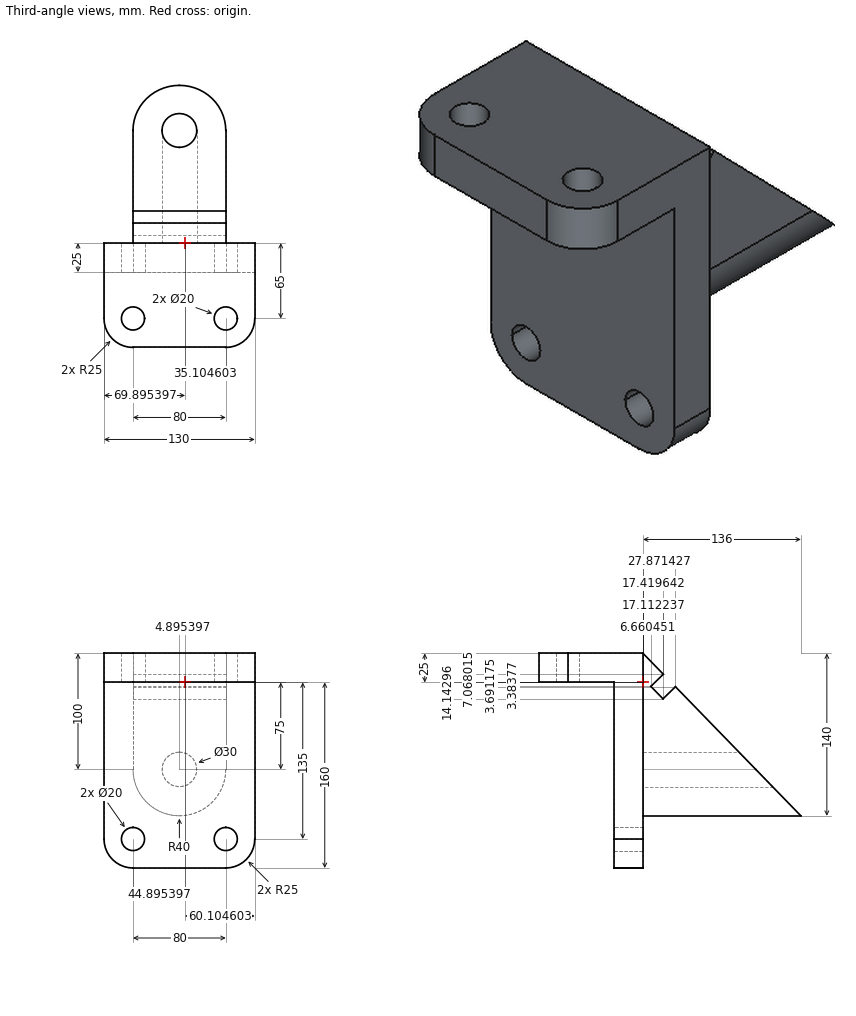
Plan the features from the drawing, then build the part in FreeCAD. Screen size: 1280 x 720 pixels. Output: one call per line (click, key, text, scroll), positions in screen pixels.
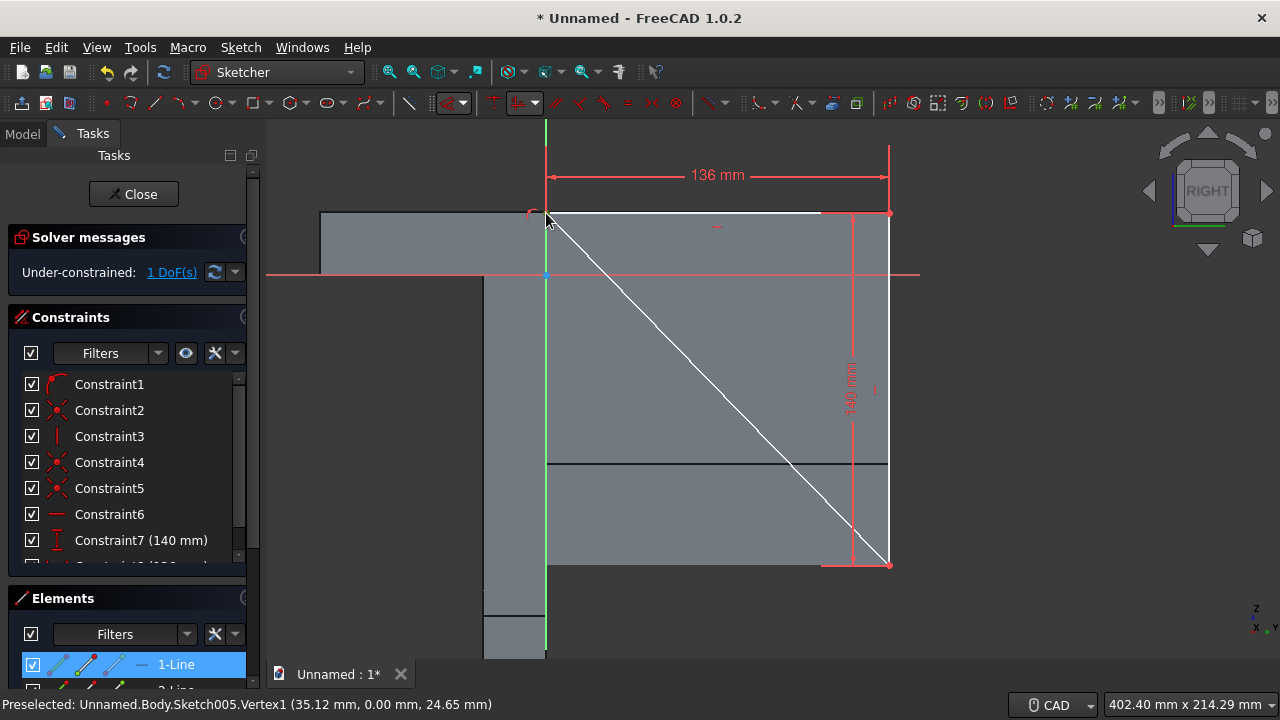
key(i)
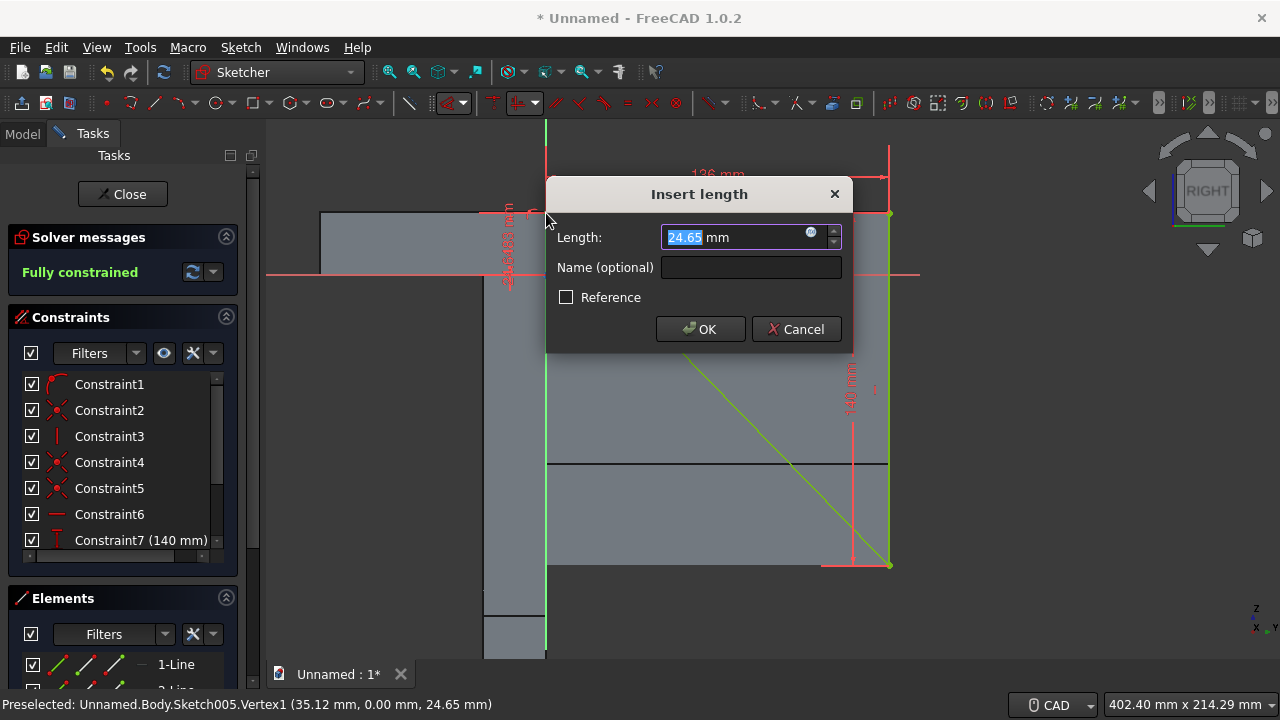
text(25)
key(Return)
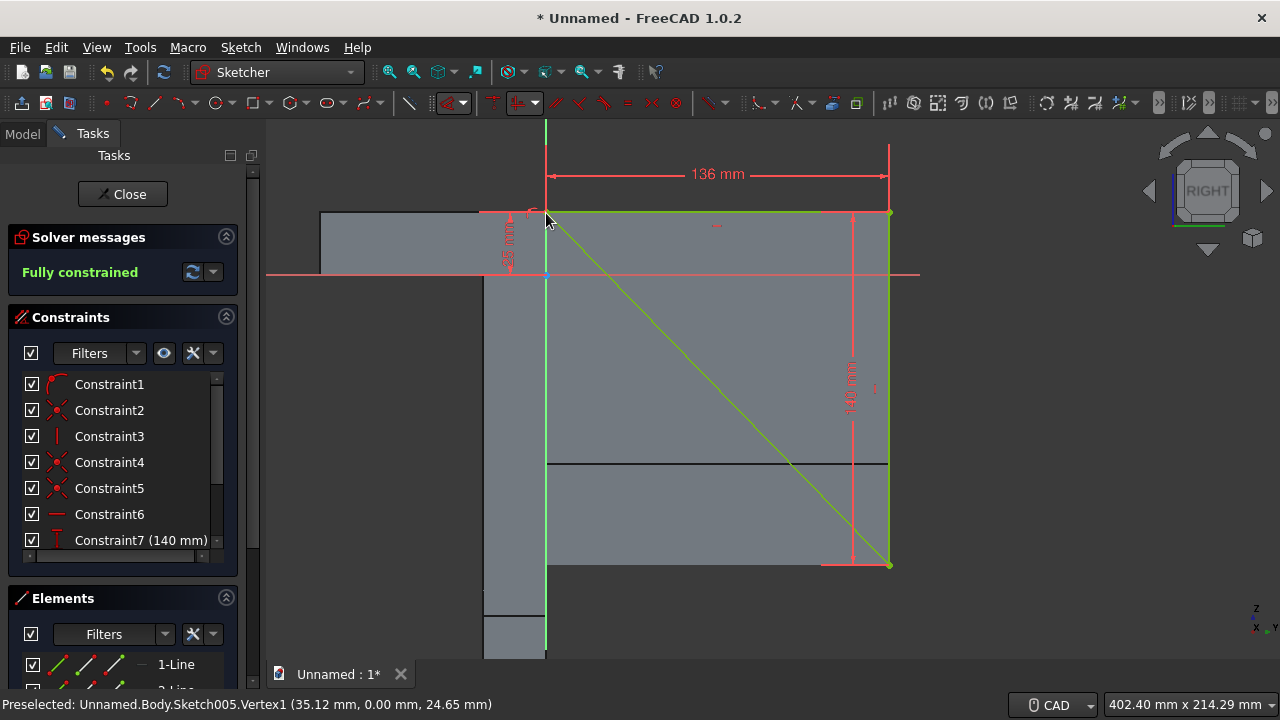
click(123, 194)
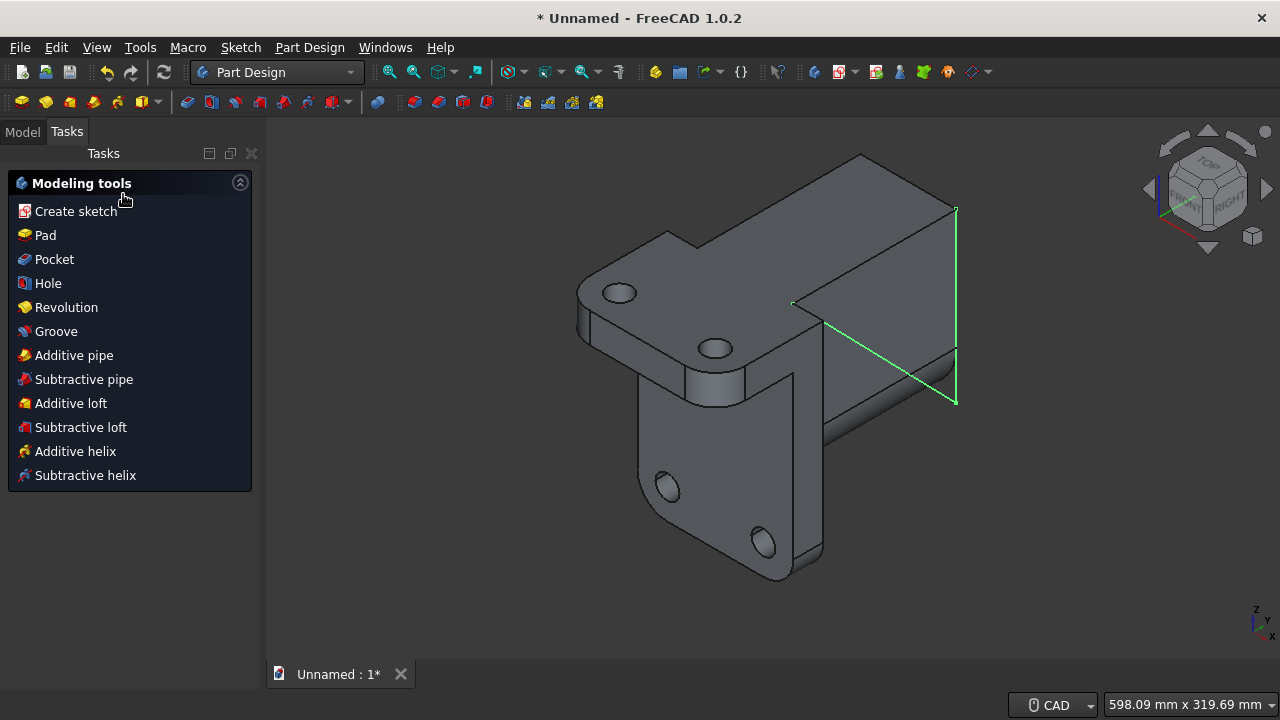
click(188, 102)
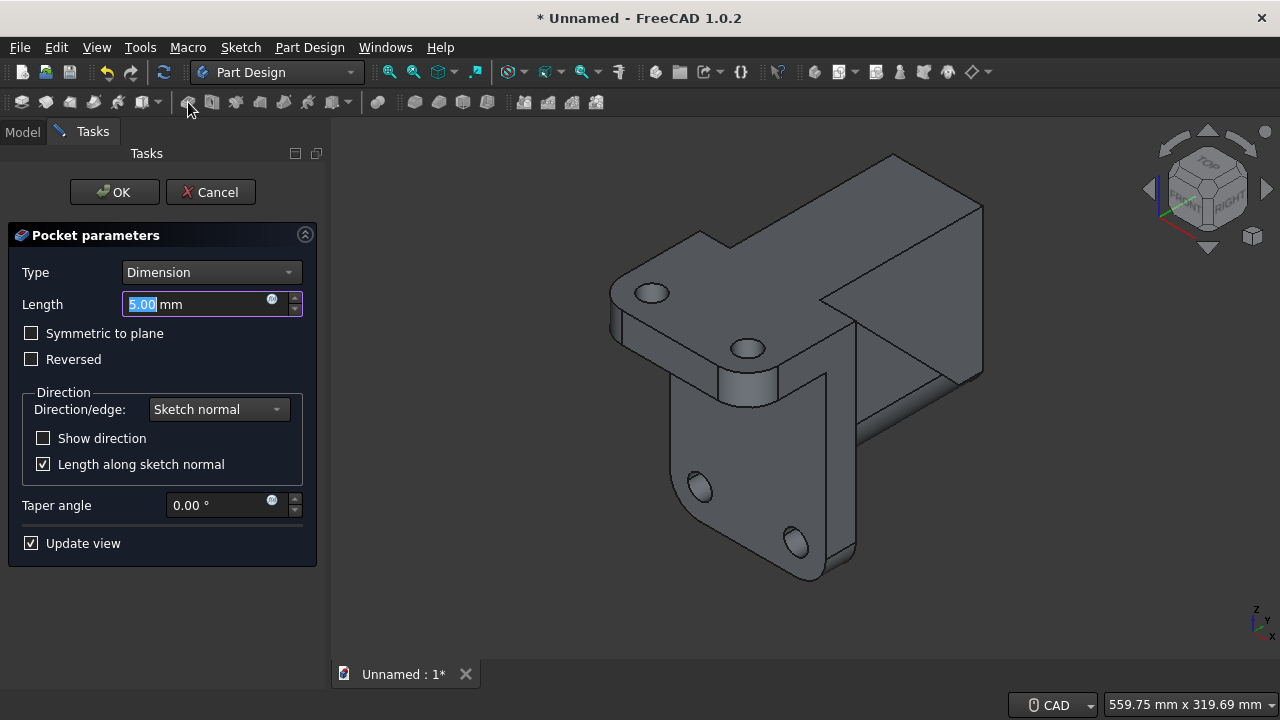
text(136)
key(Tab)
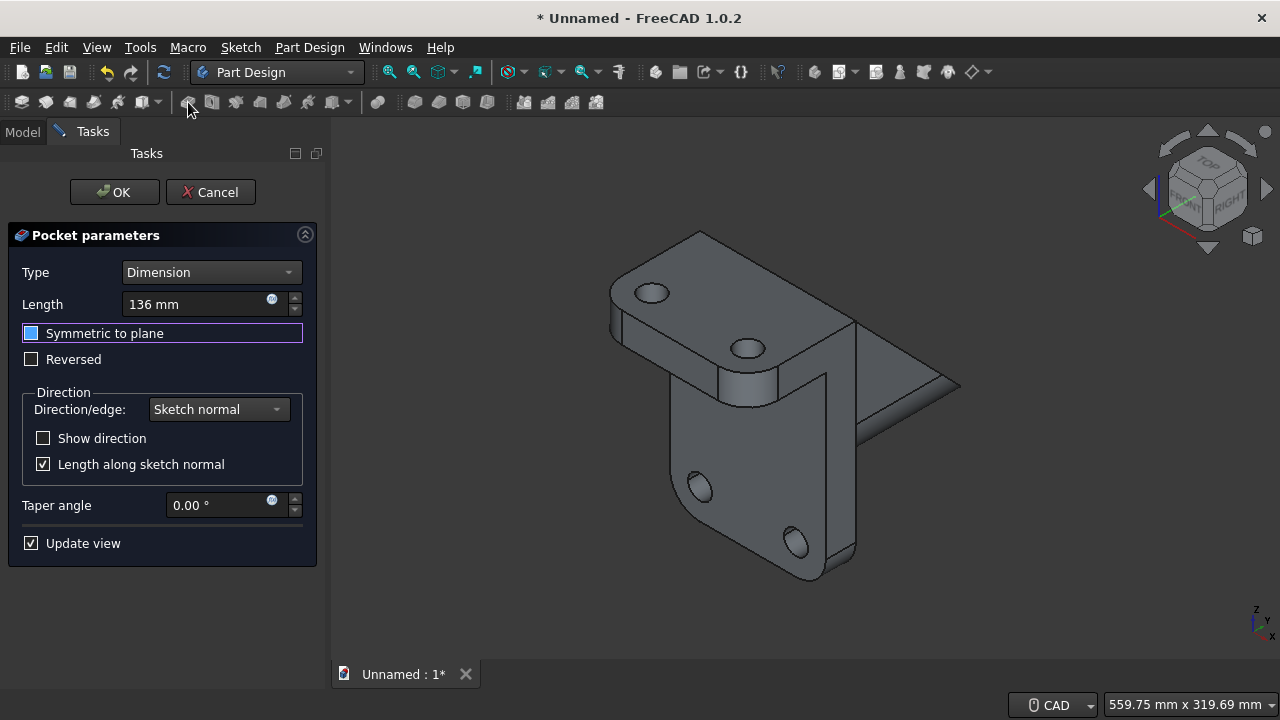
click(115, 192)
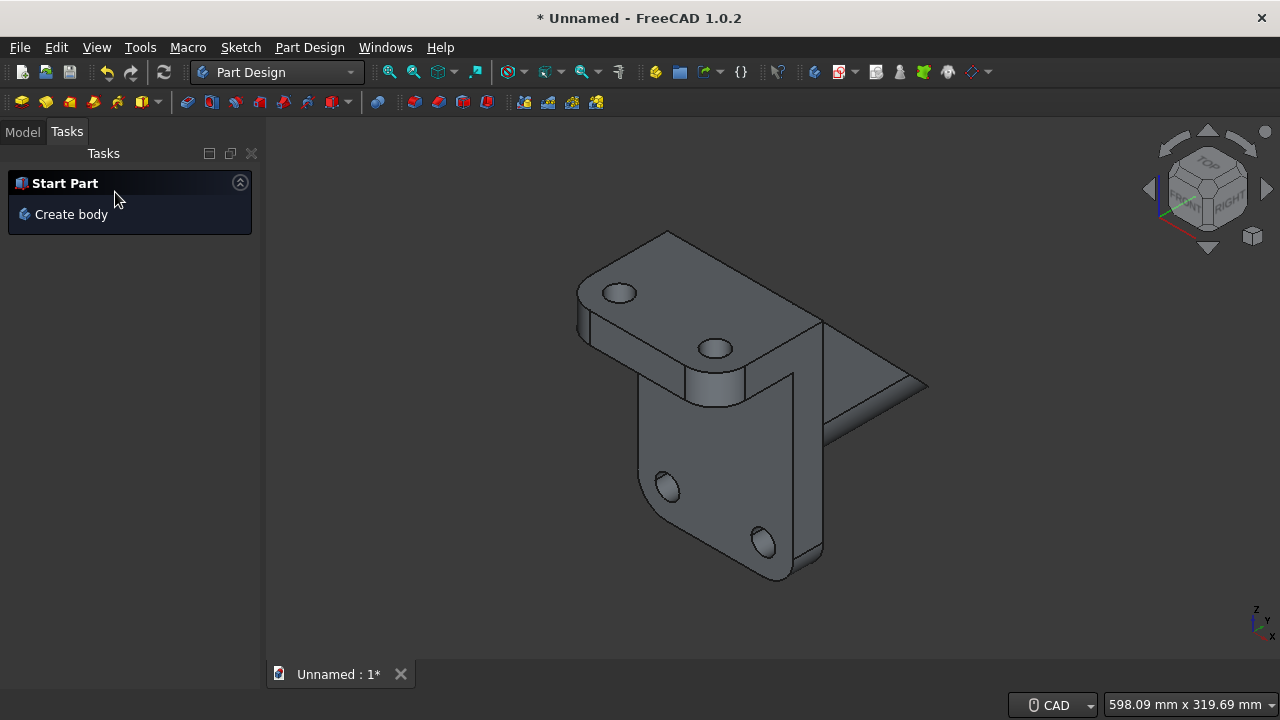
click(835, 387)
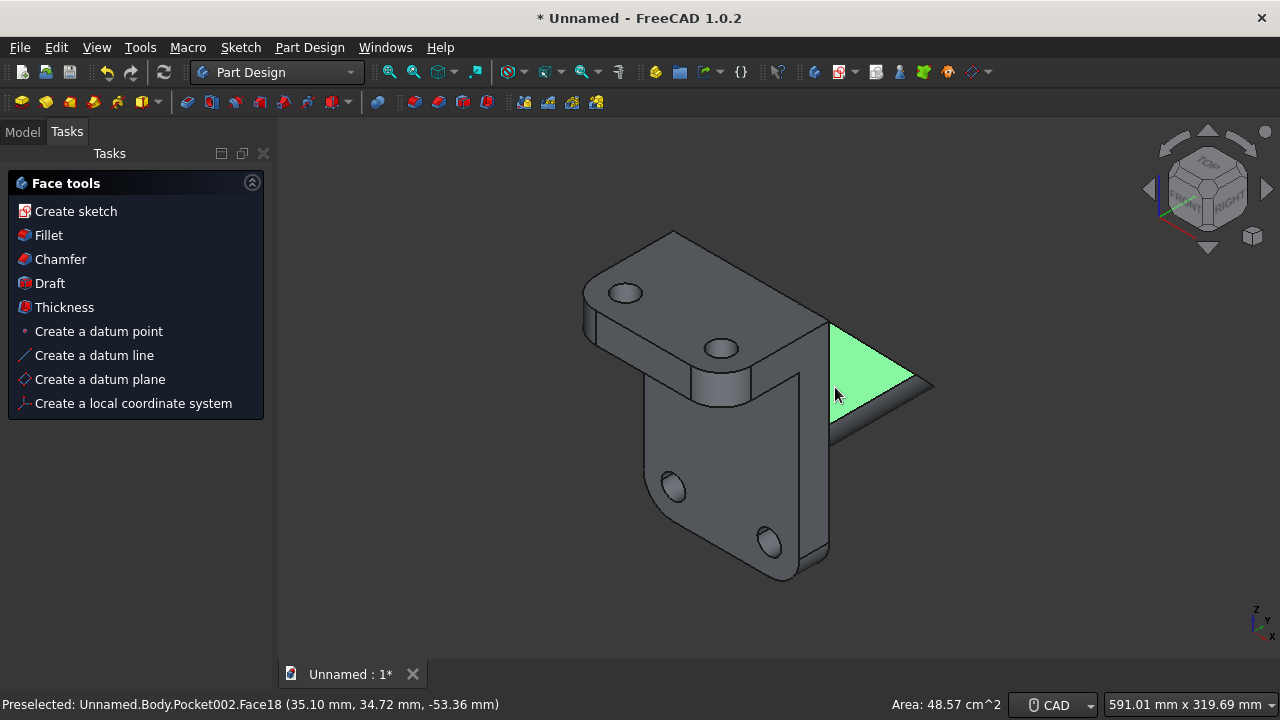
click(840, 72)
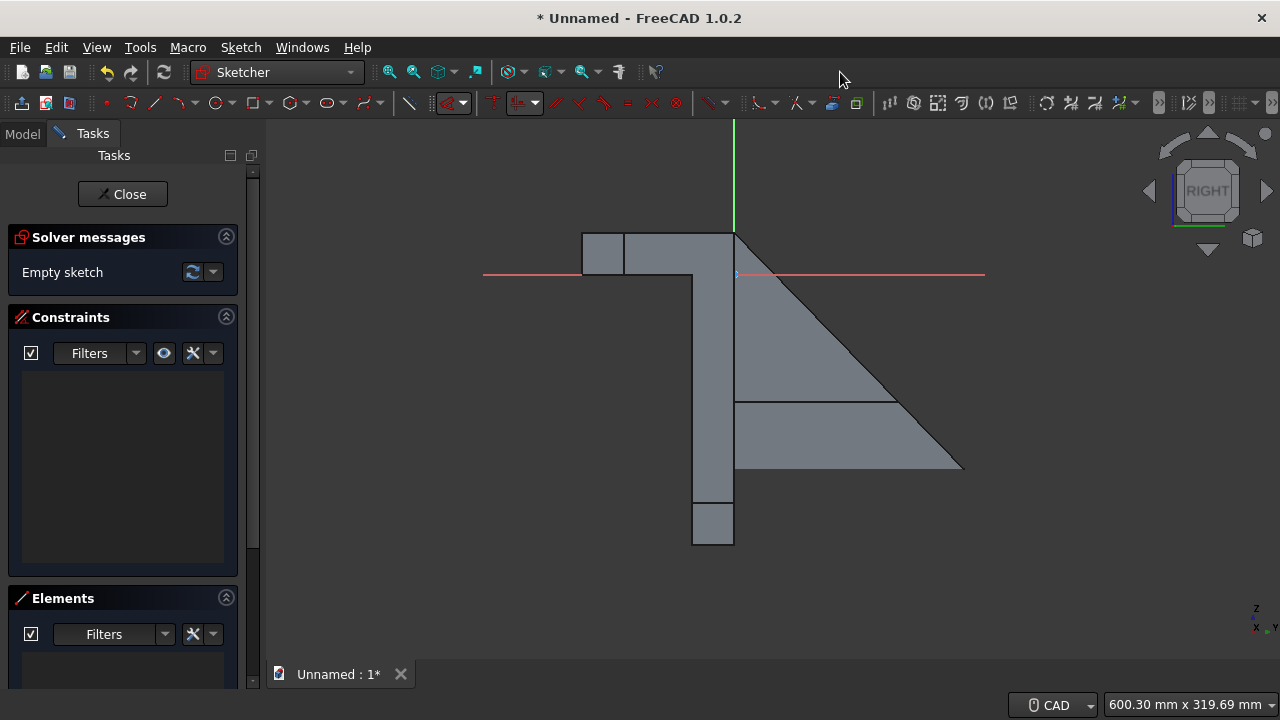
click(70, 104)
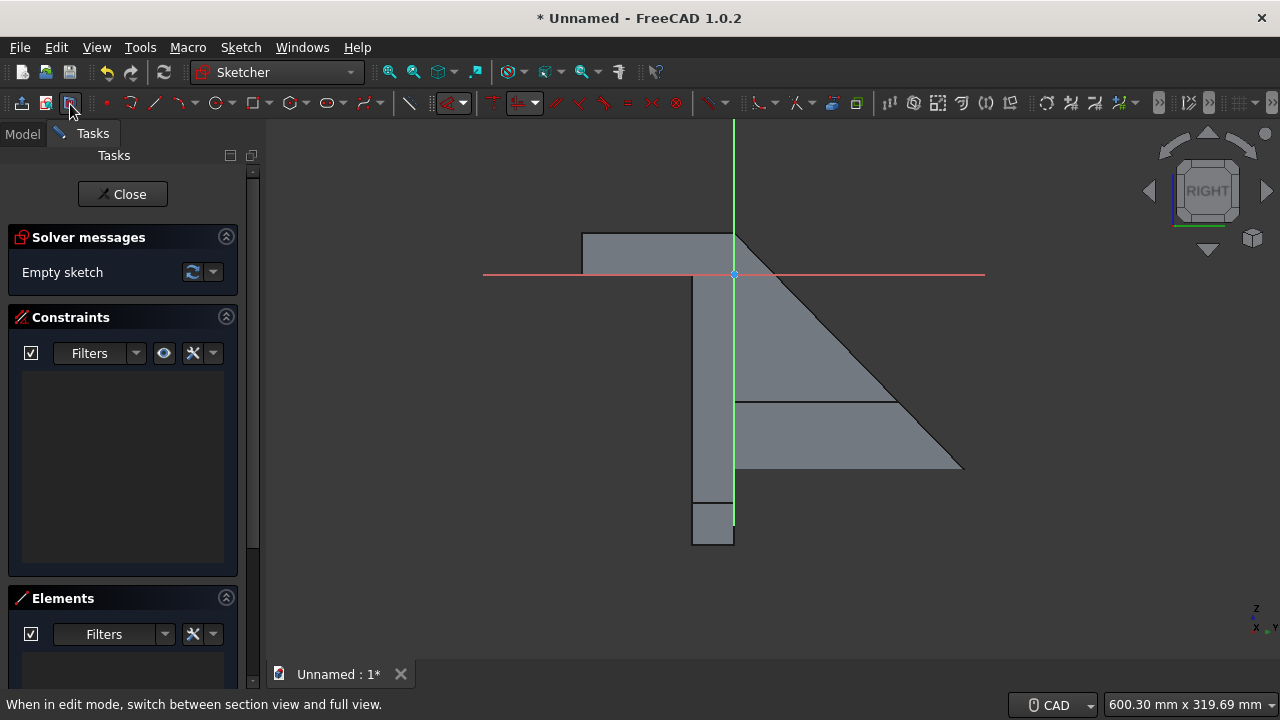
scroll(764, 267, up, 11)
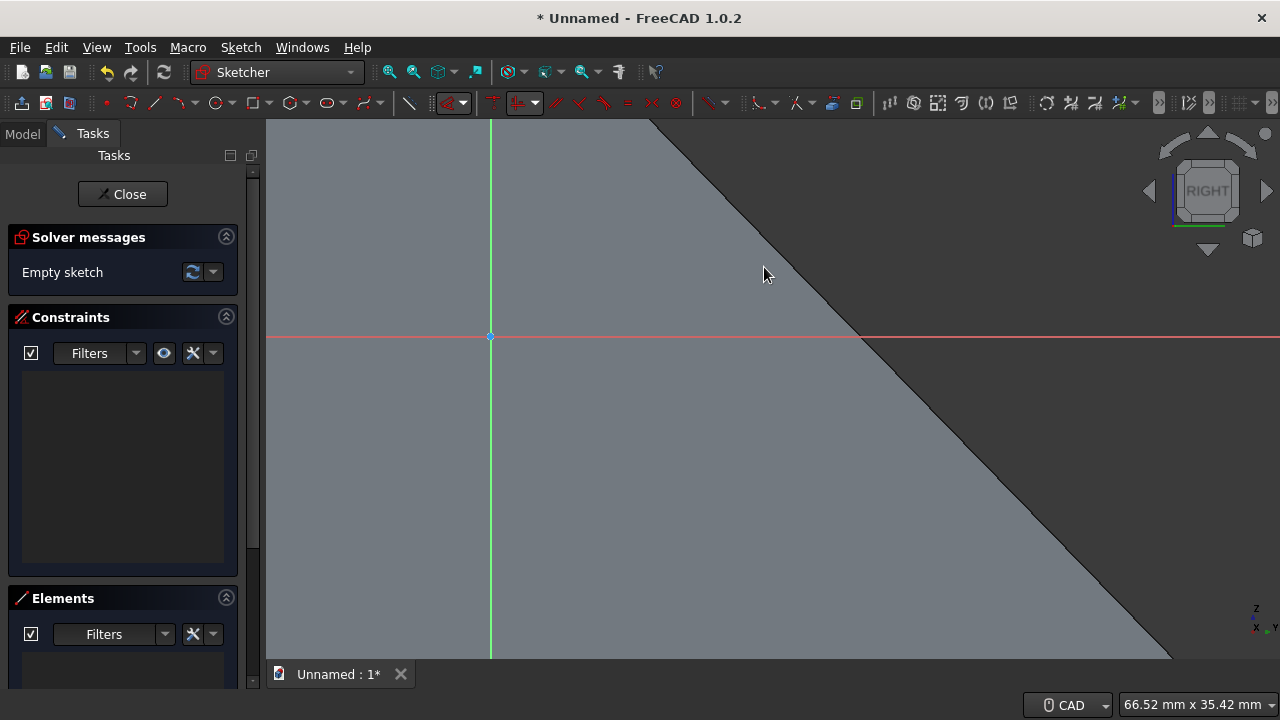
click(132, 104)